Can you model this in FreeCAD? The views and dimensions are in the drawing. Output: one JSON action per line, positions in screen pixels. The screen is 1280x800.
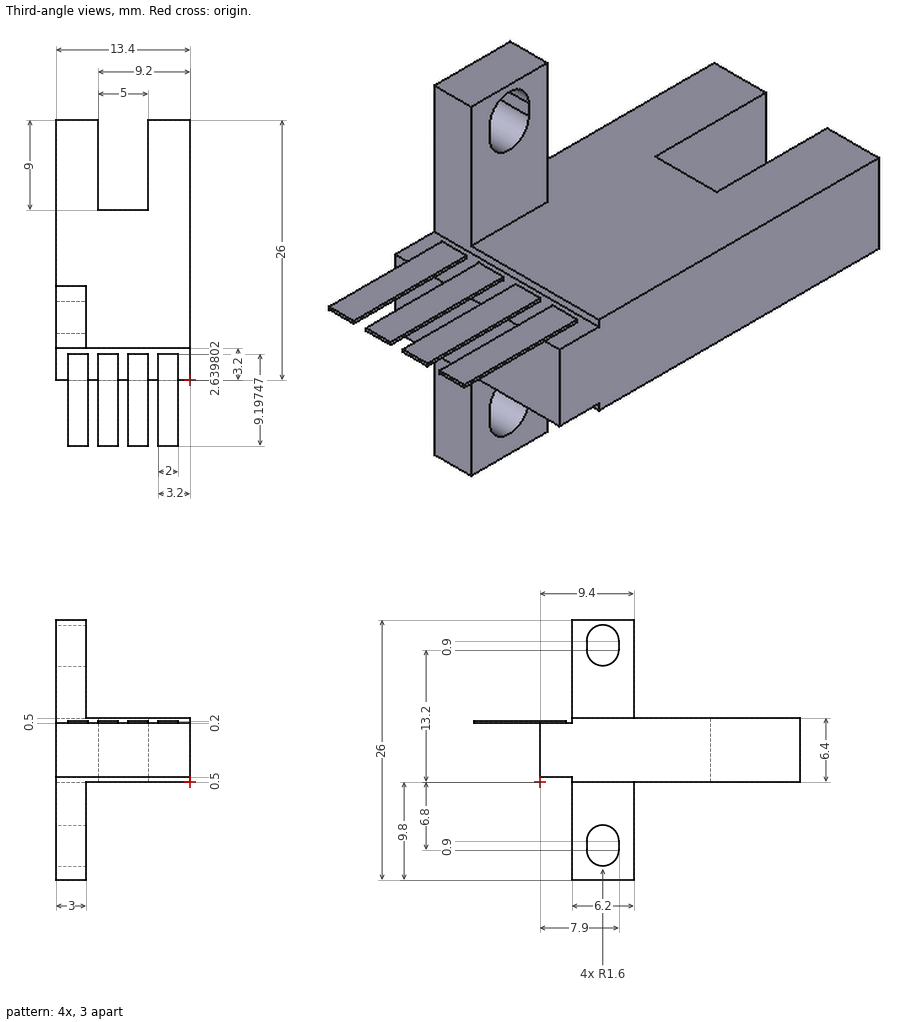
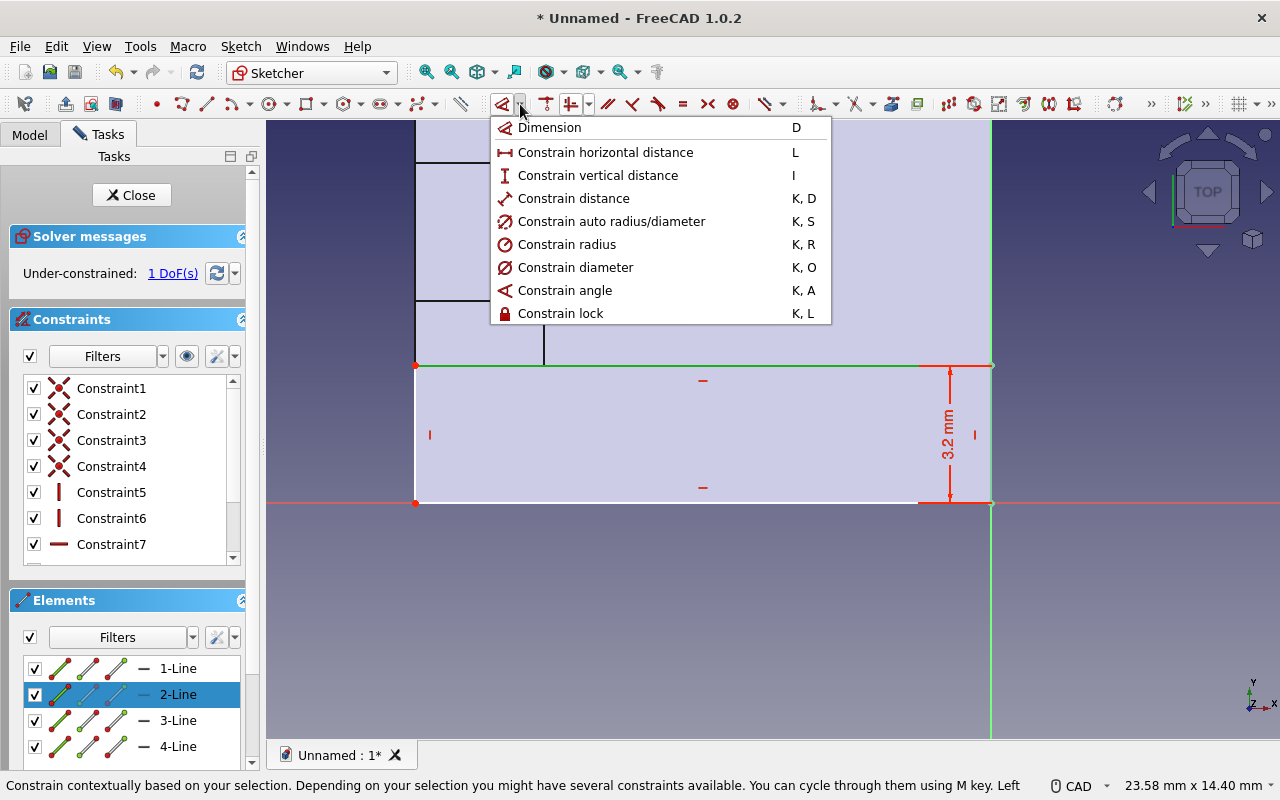
{"action": "left_click", "coordinate": [661, 152]}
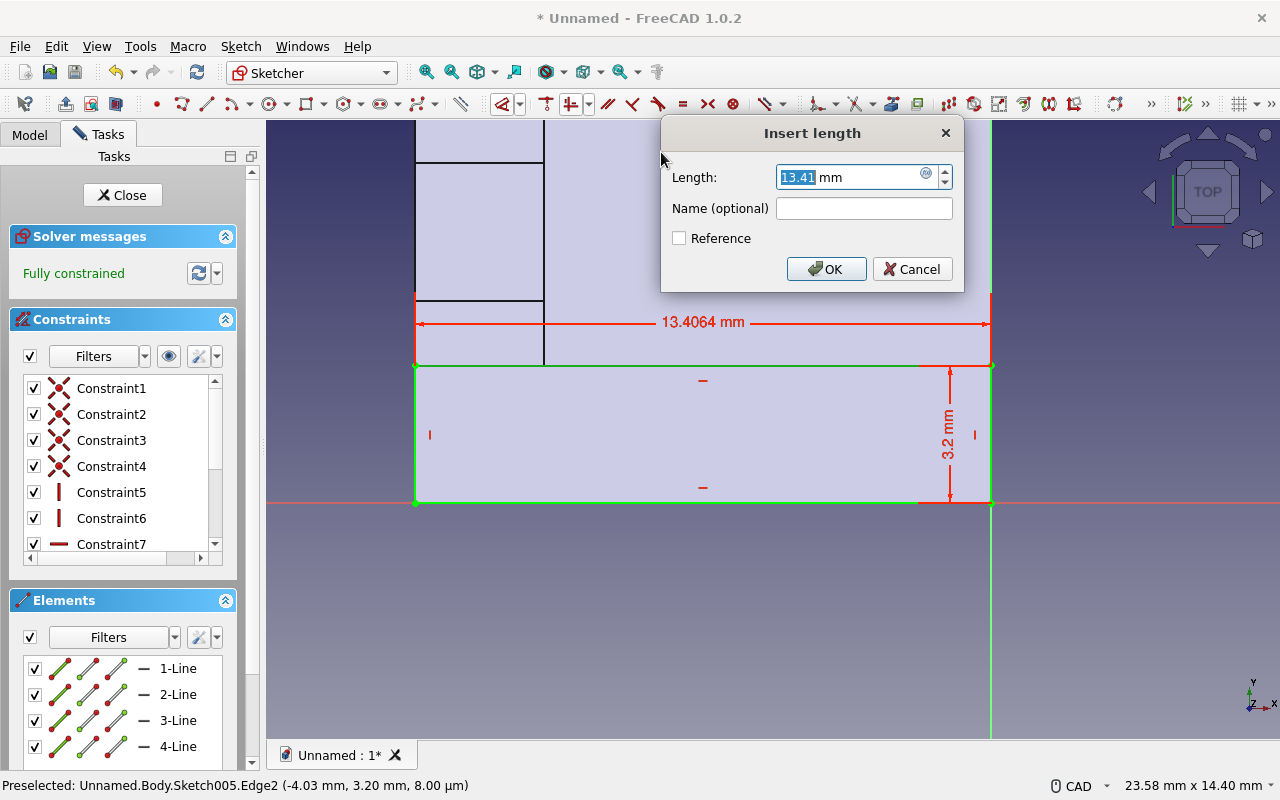
{"action": "type", "text": "13.4"}
{"action": "key", "text": "Return"}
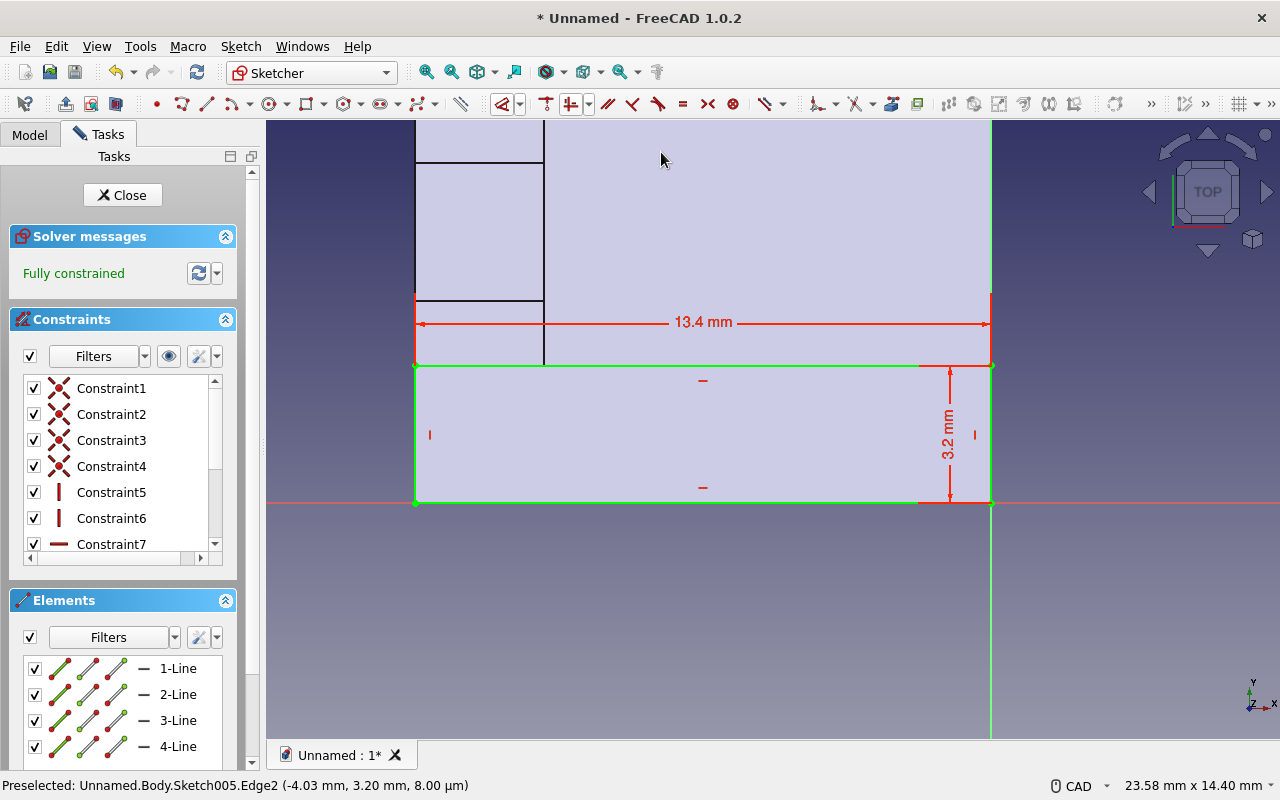
{"action": "left_click", "coordinate": [123, 195]}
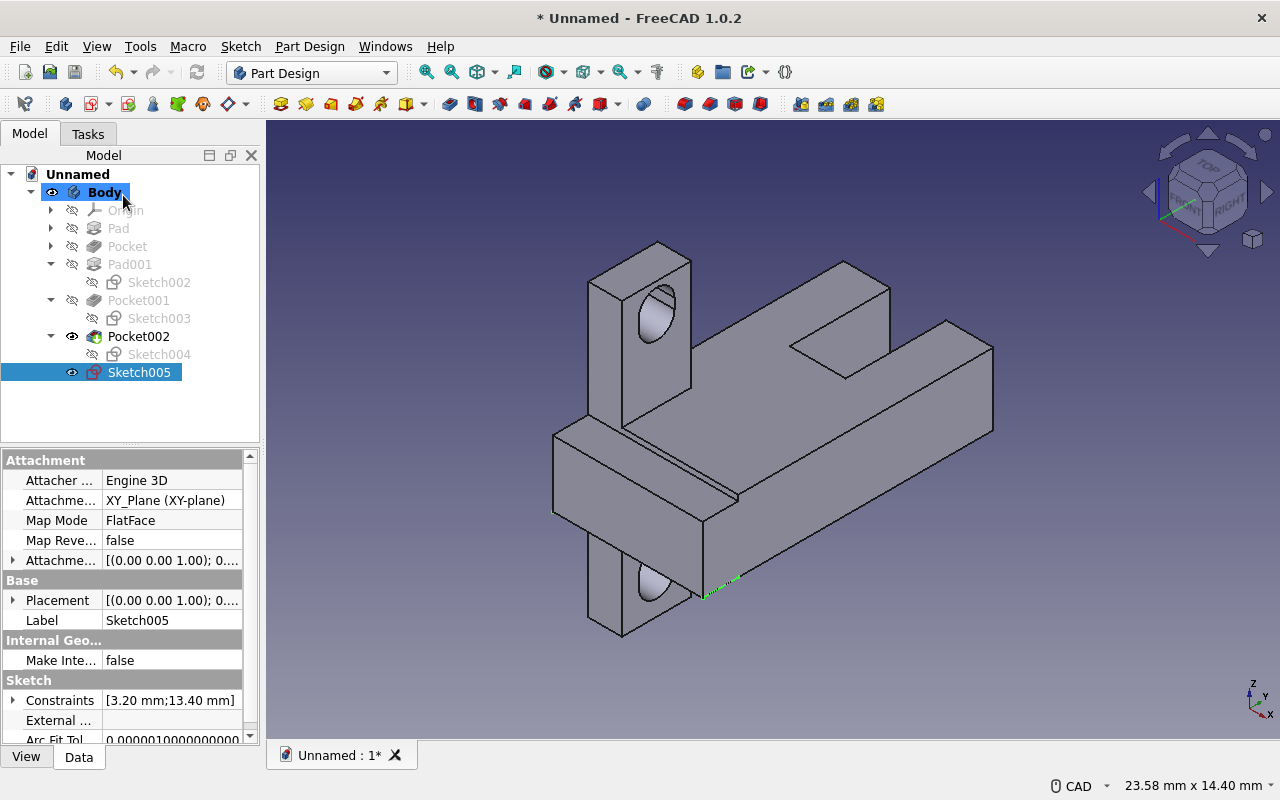
{"action": "left_click", "coordinate": [450, 104]}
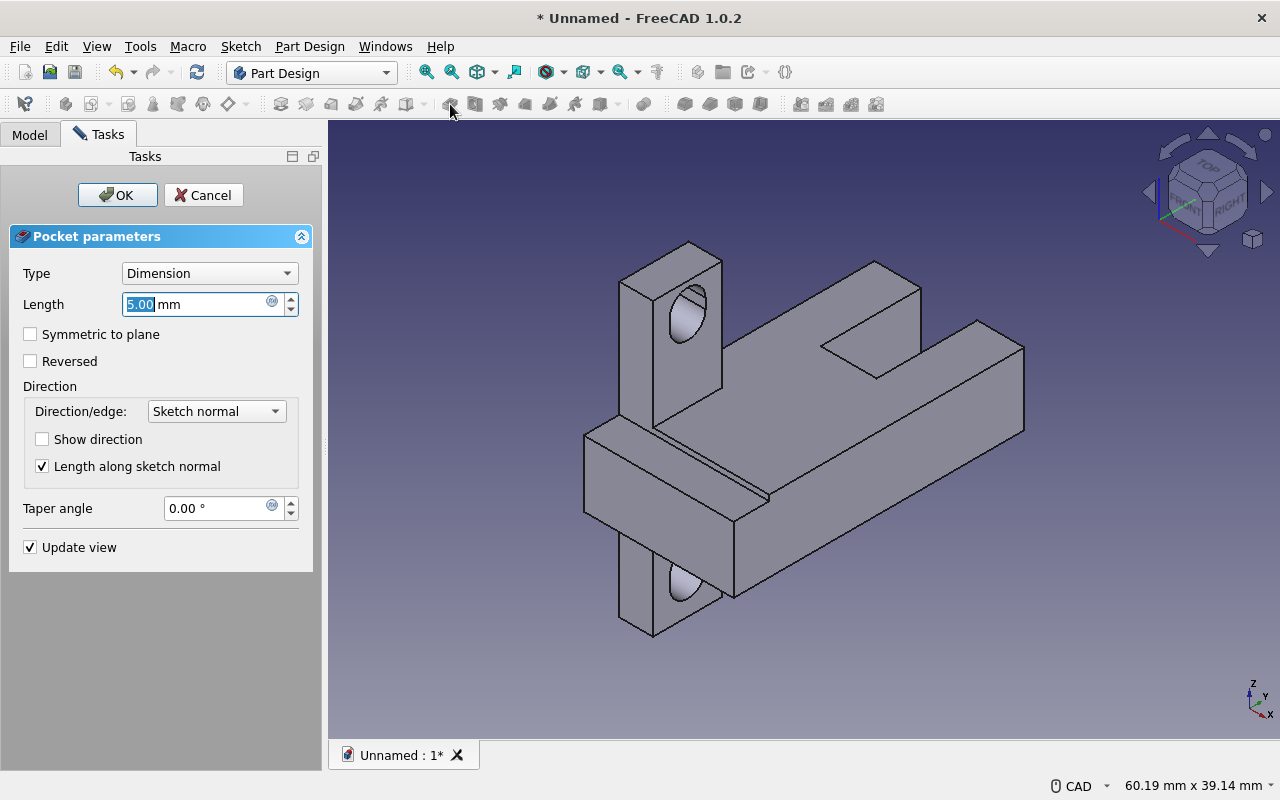
{"action": "type", "text": "0.5"}
{"action": "key", "text": "Tab"}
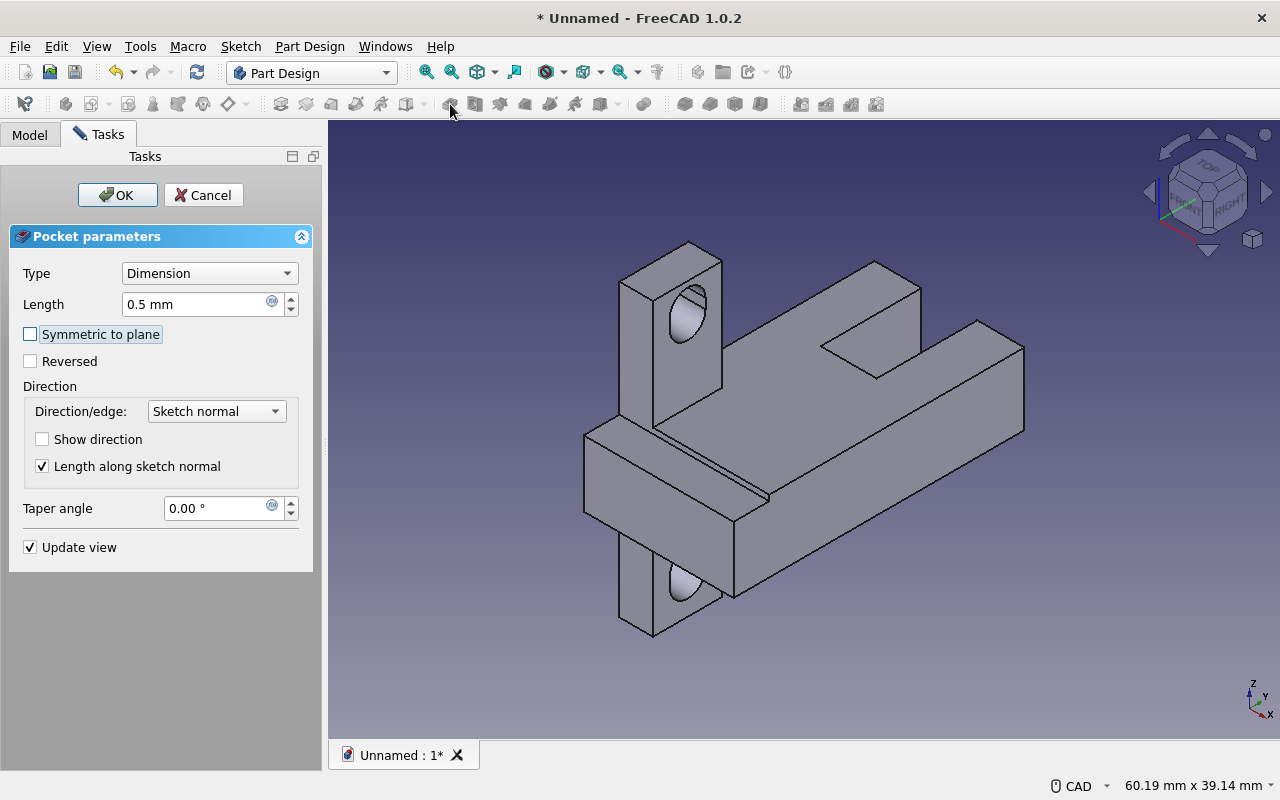
{"action": "left_click", "coordinate": [31, 361]}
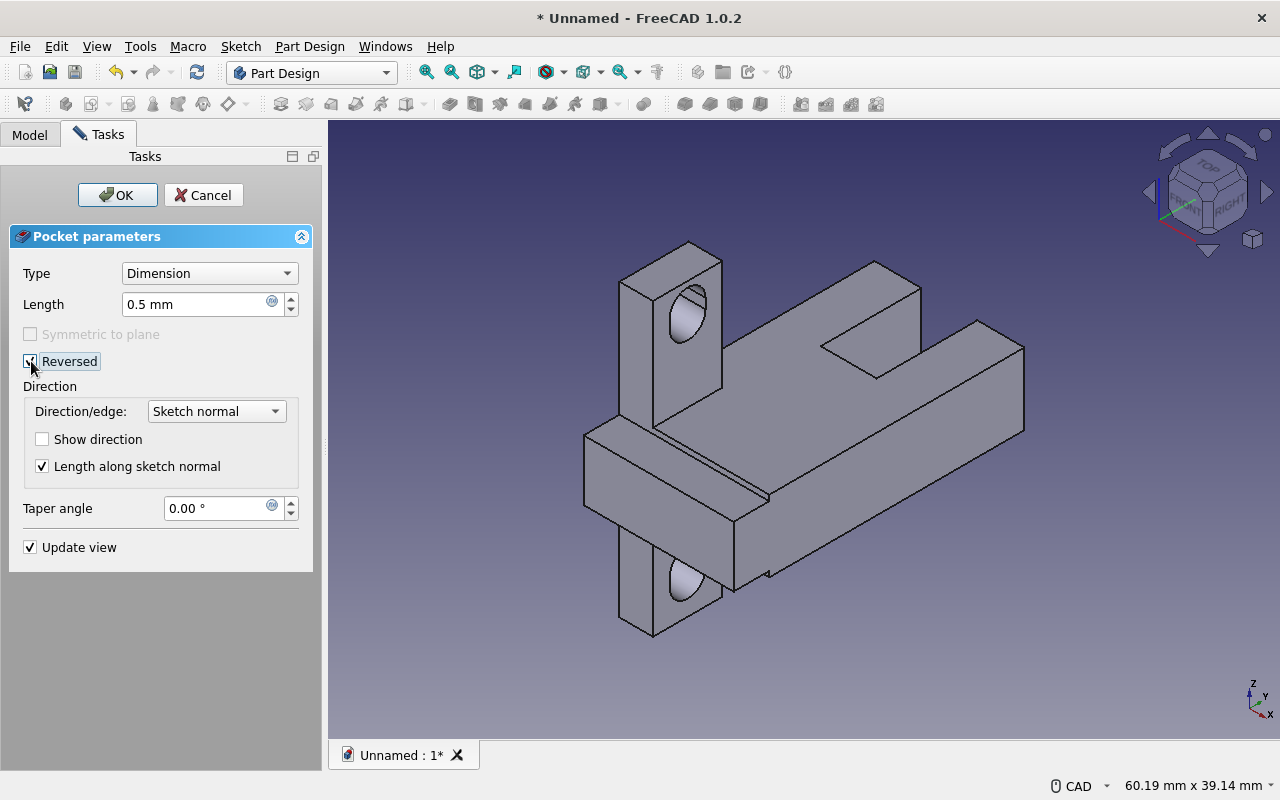
{"action": "left_click", "coordinate": [118, 195]}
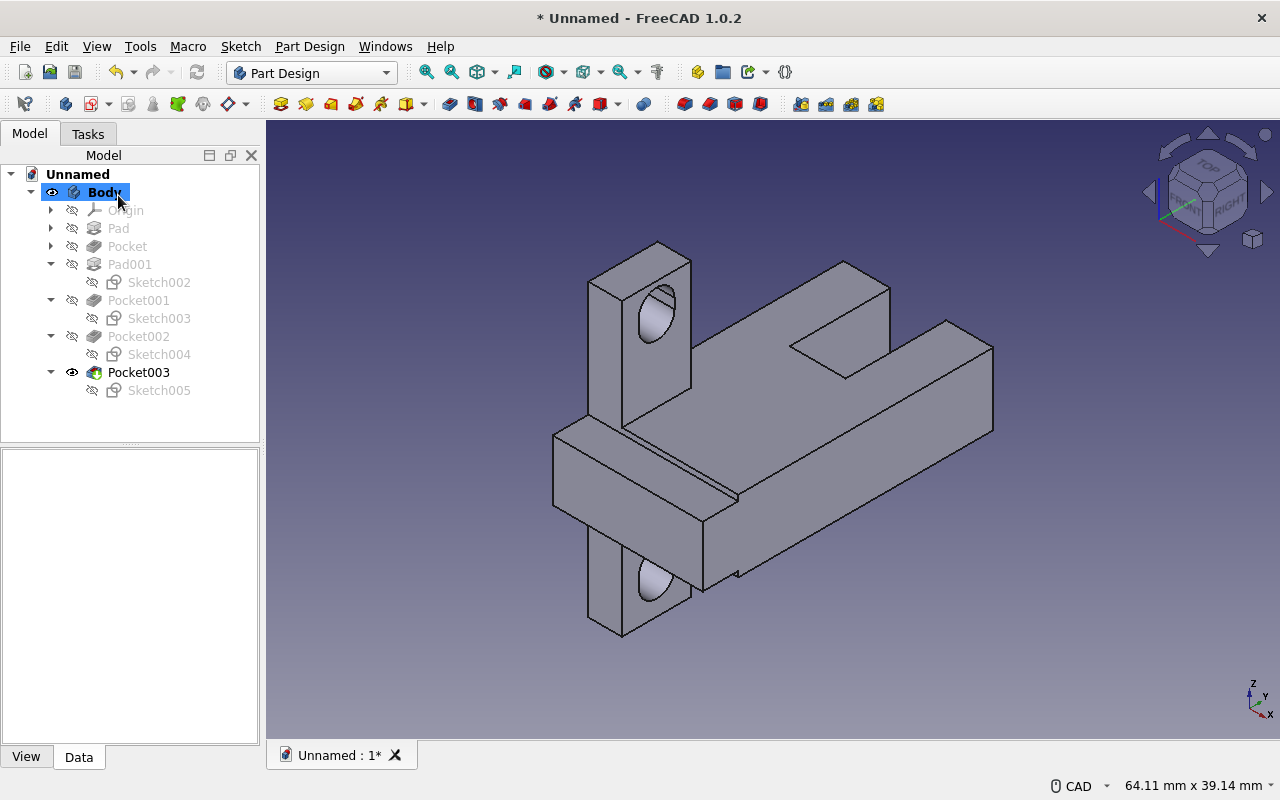
{"action": "left_click", "coordinate": [688, 492]}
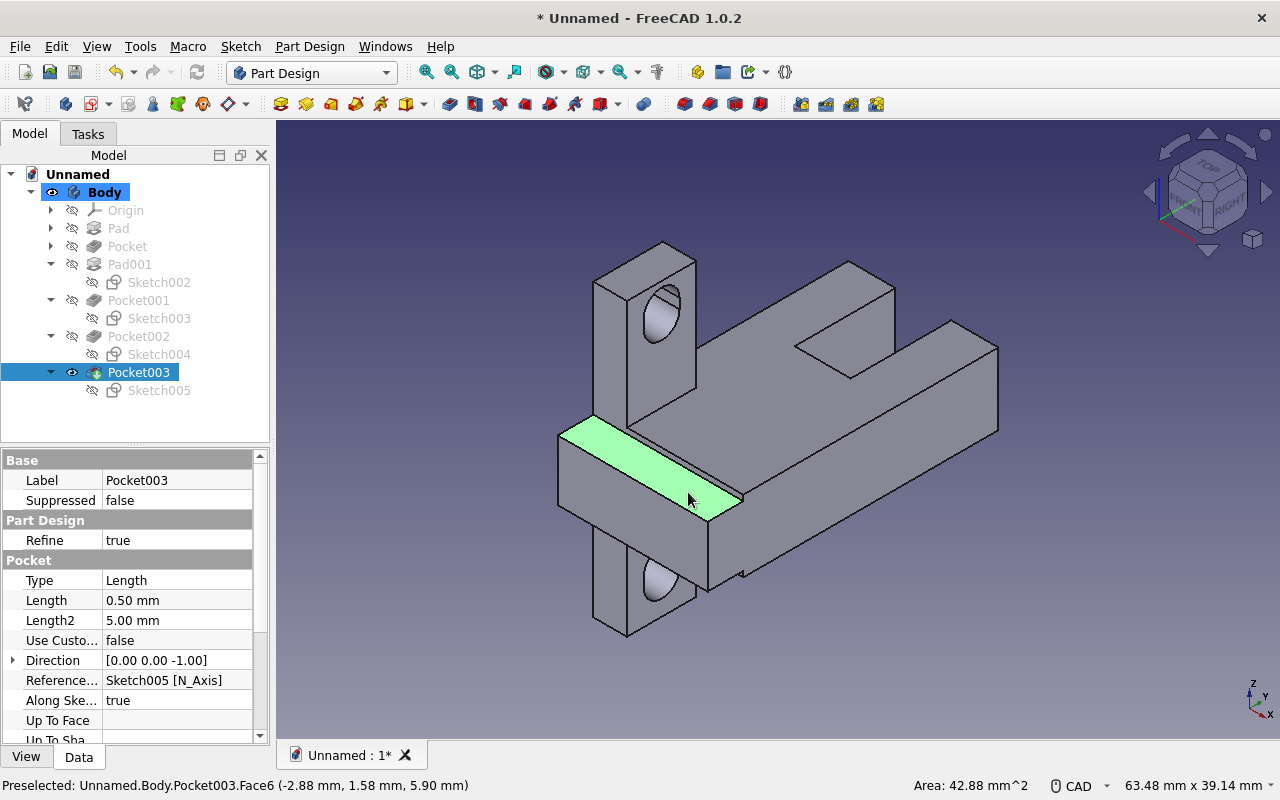
{"action": "left_click", "coordinate": [90, 104]}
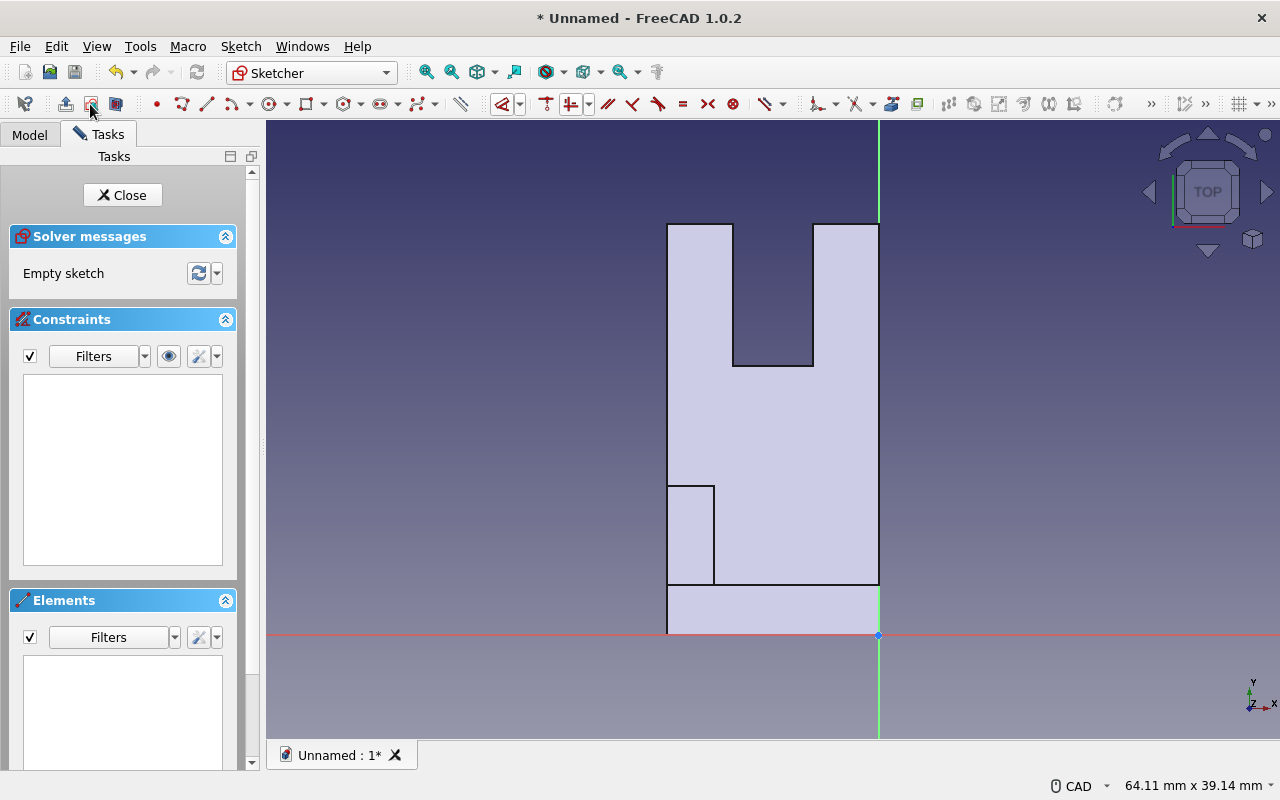
{"action": "left_click", "coordinate": [116, 104]}